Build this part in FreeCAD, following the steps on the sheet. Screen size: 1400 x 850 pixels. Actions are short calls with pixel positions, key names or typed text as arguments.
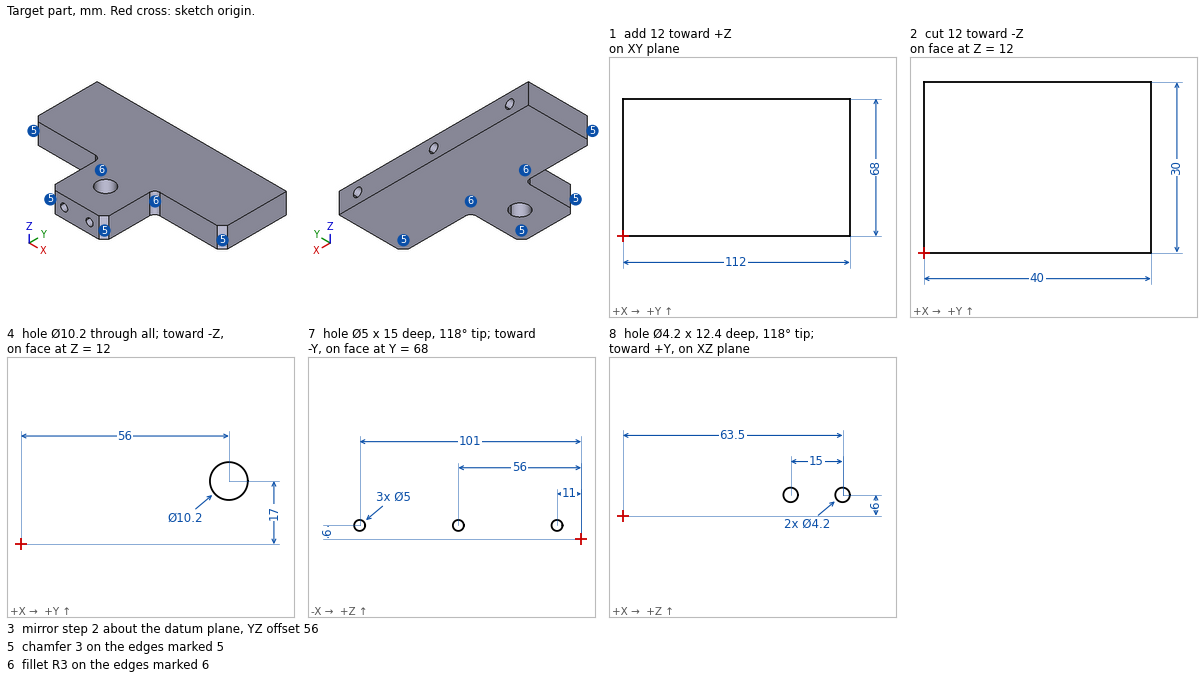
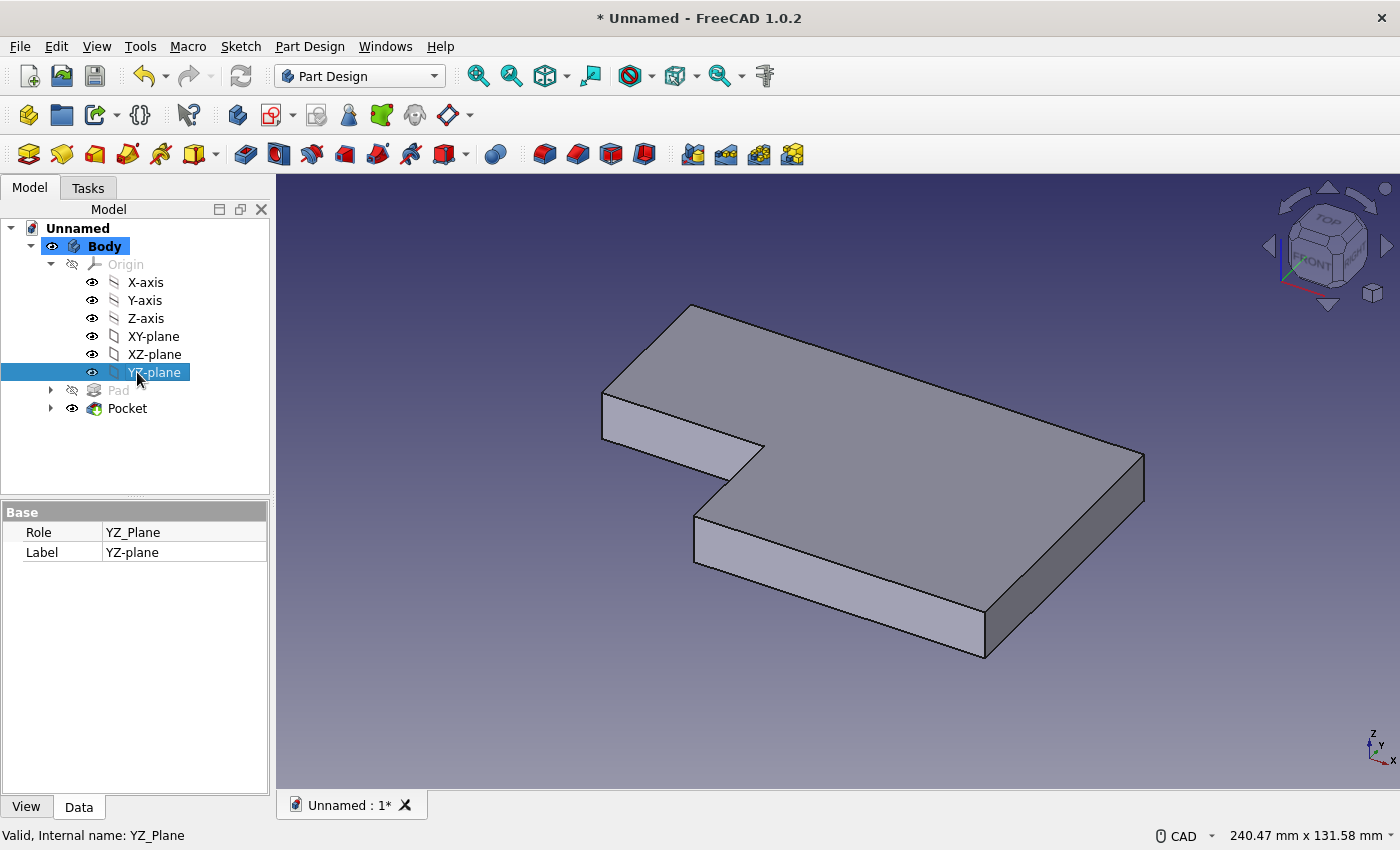
click(448, 116)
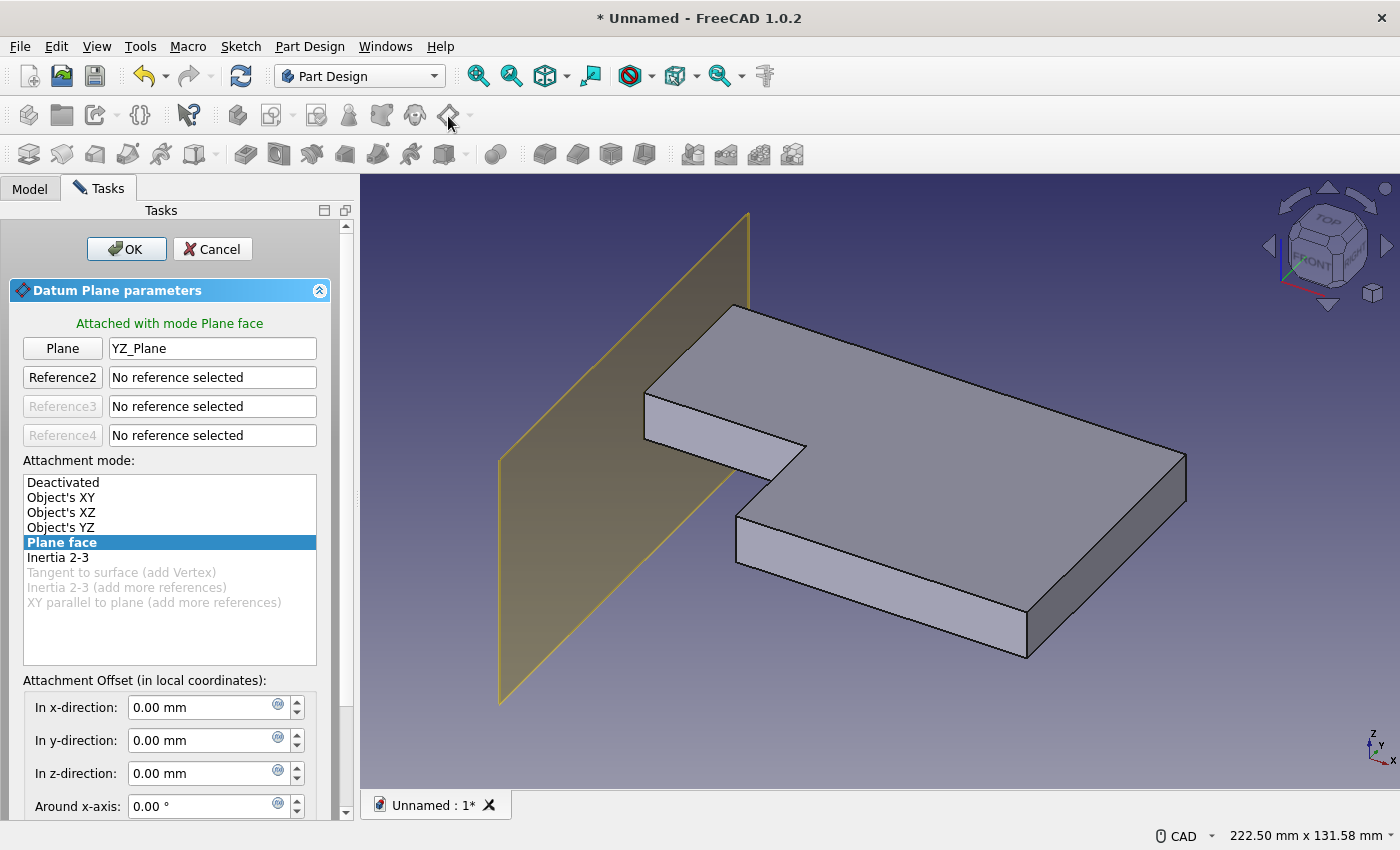
triple_click(210, 774)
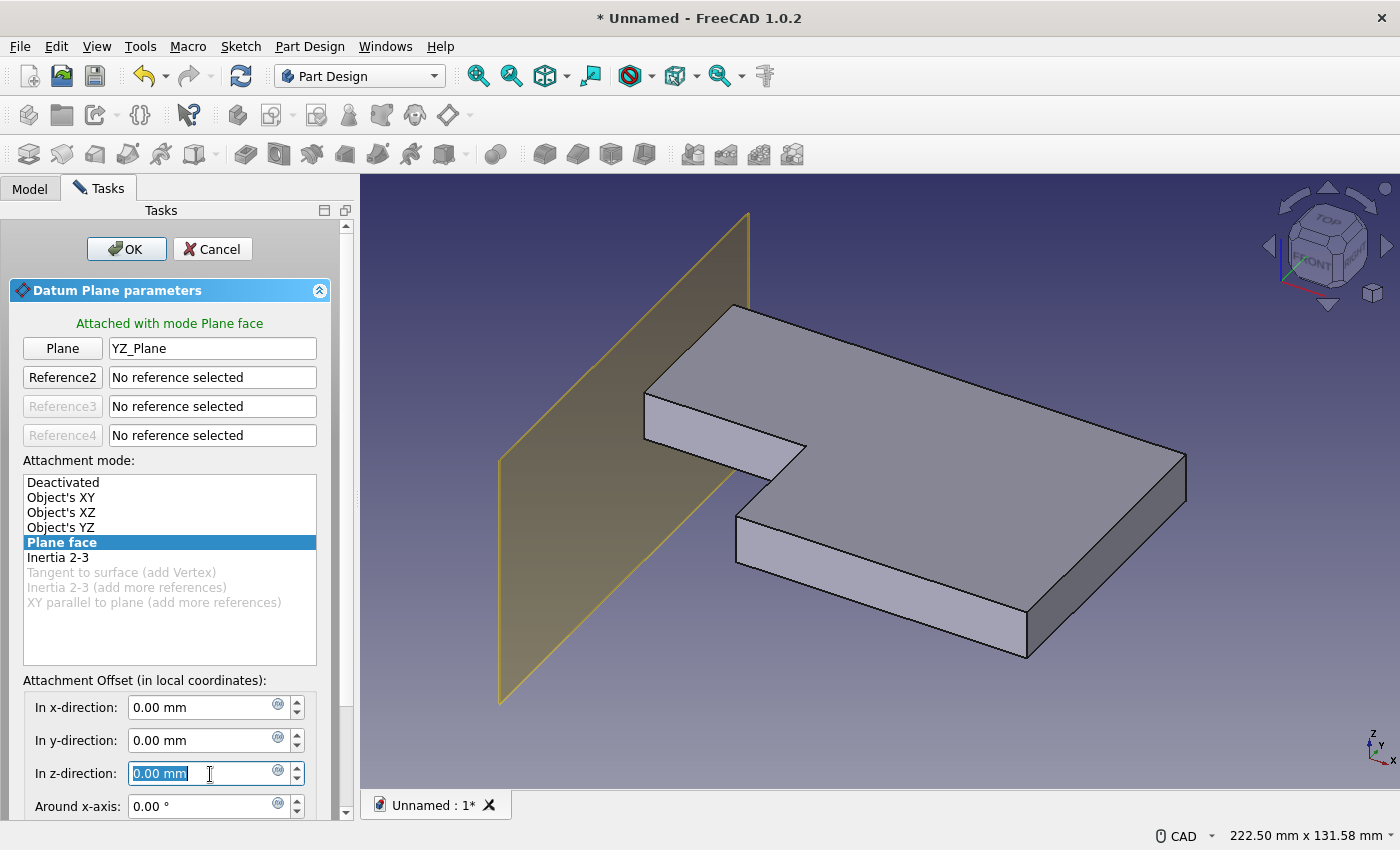
text(56)
key(Tab)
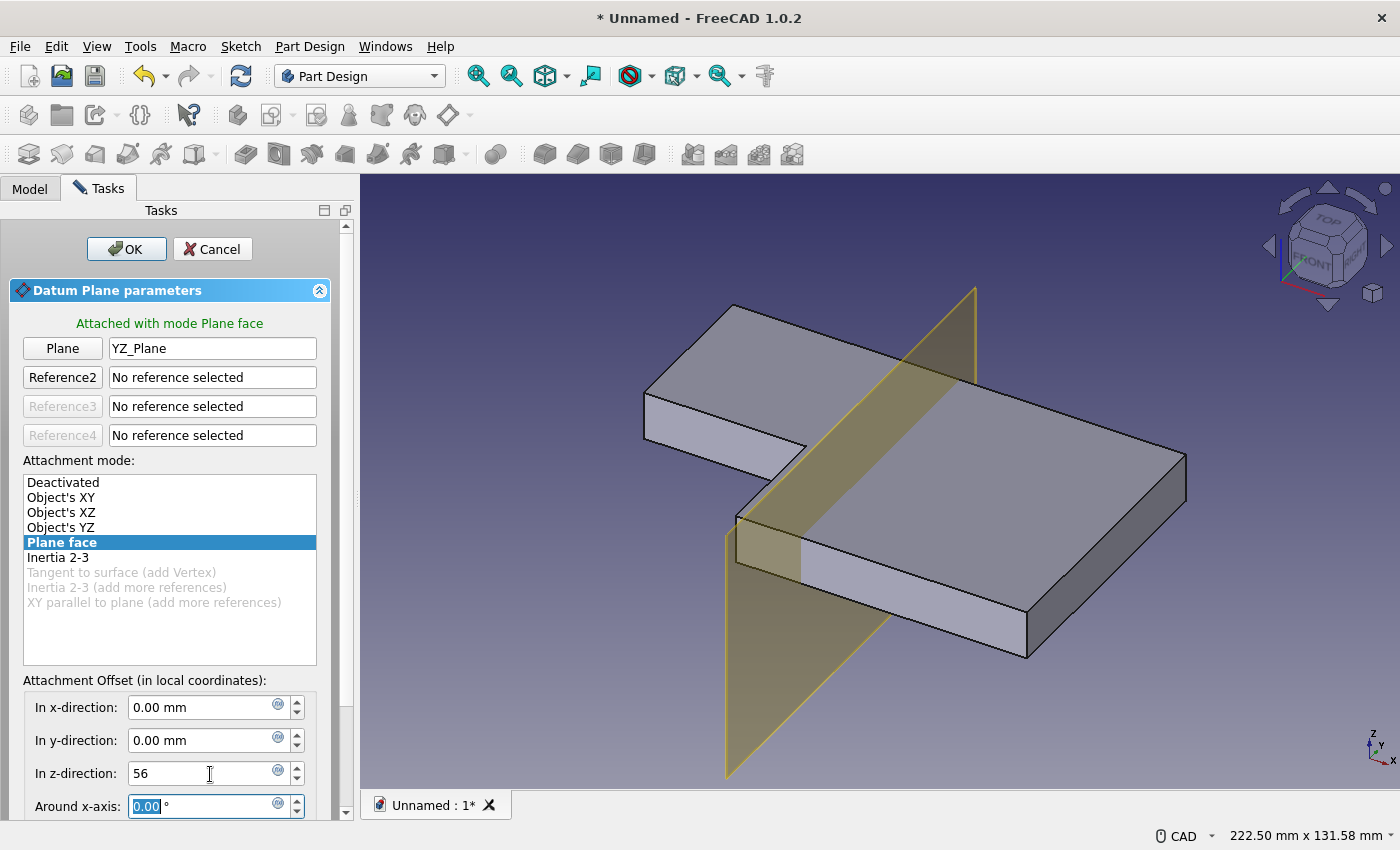
click(127, 249)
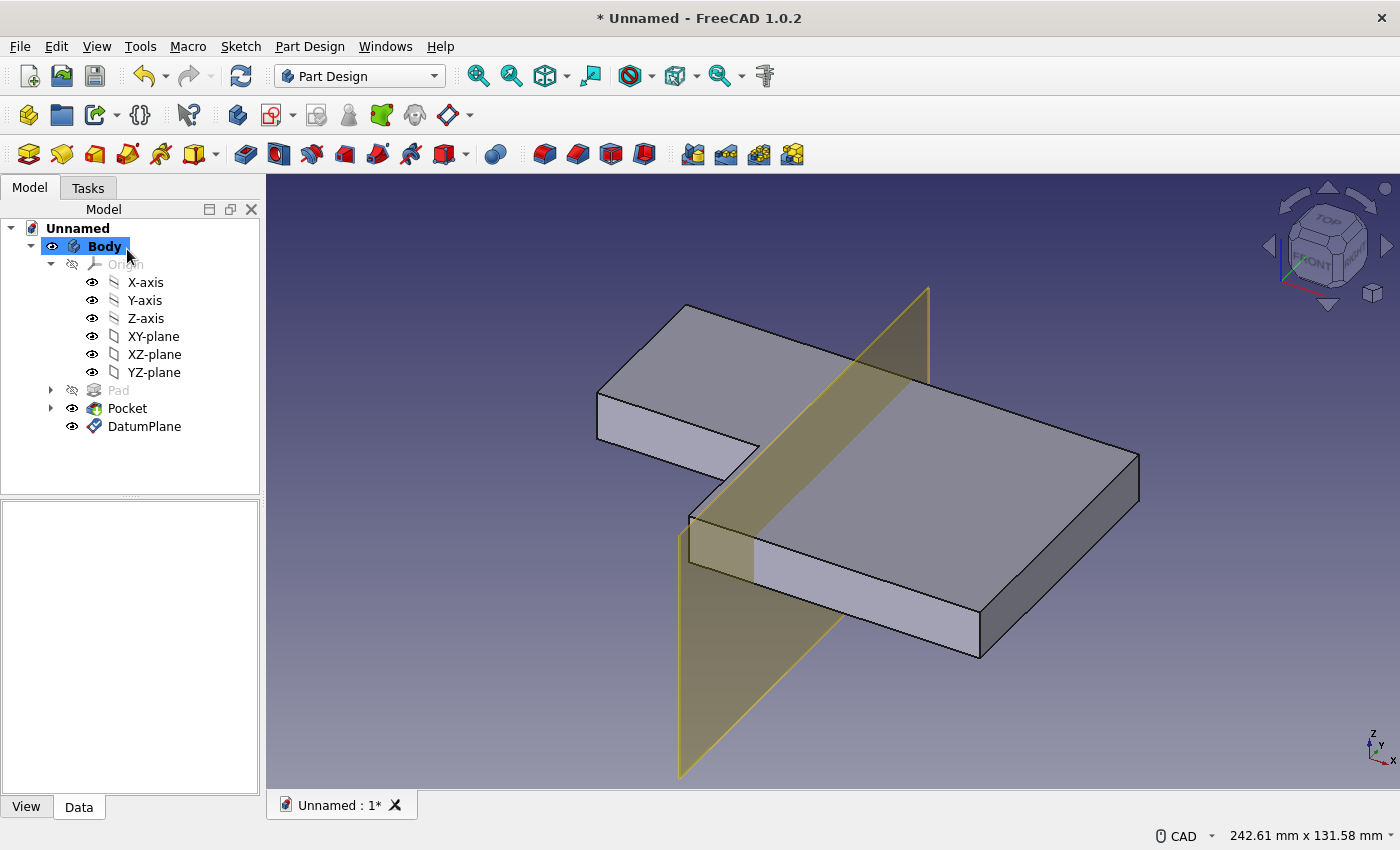
click(117, 408)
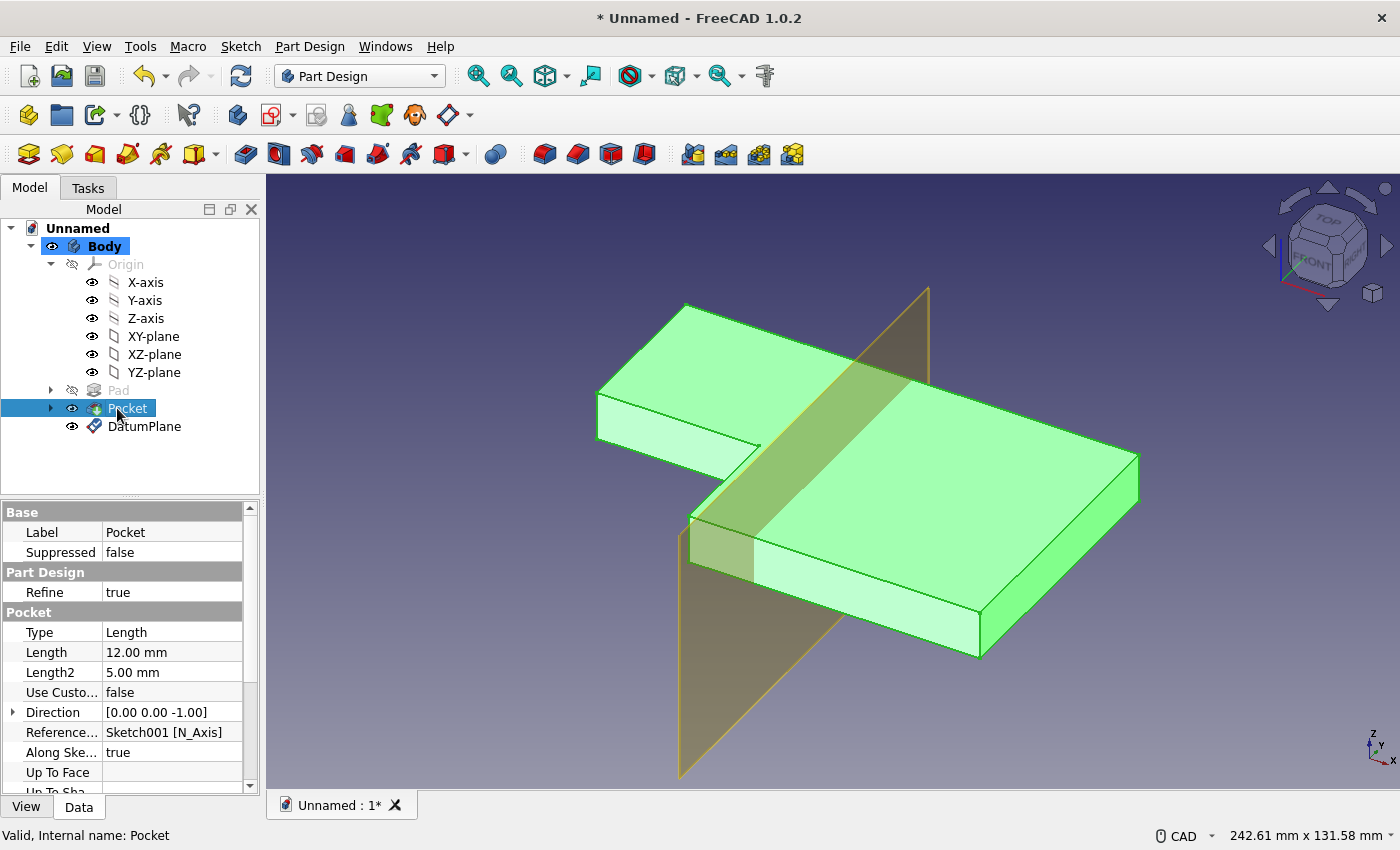
click(693, 154)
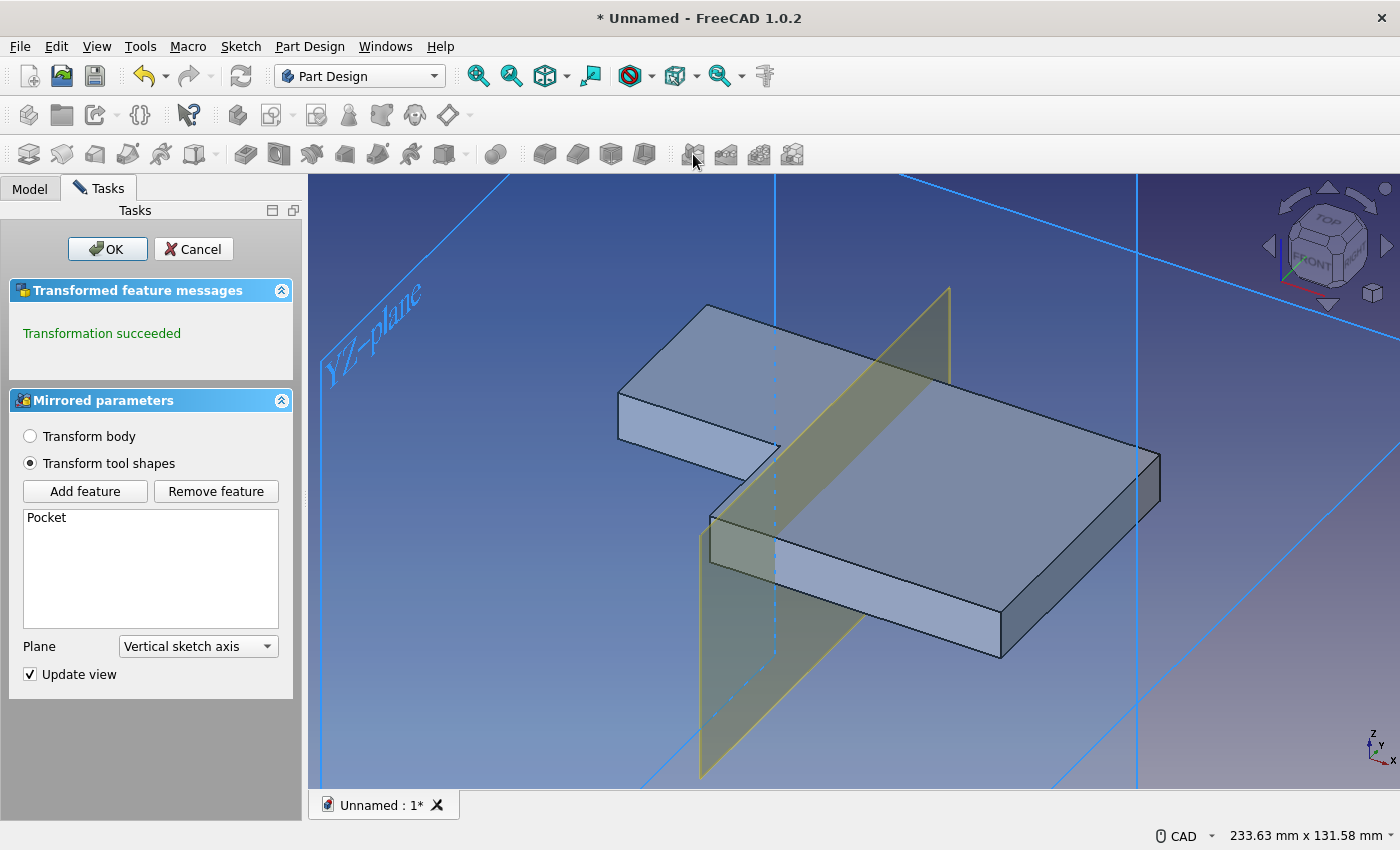
click(199, 646)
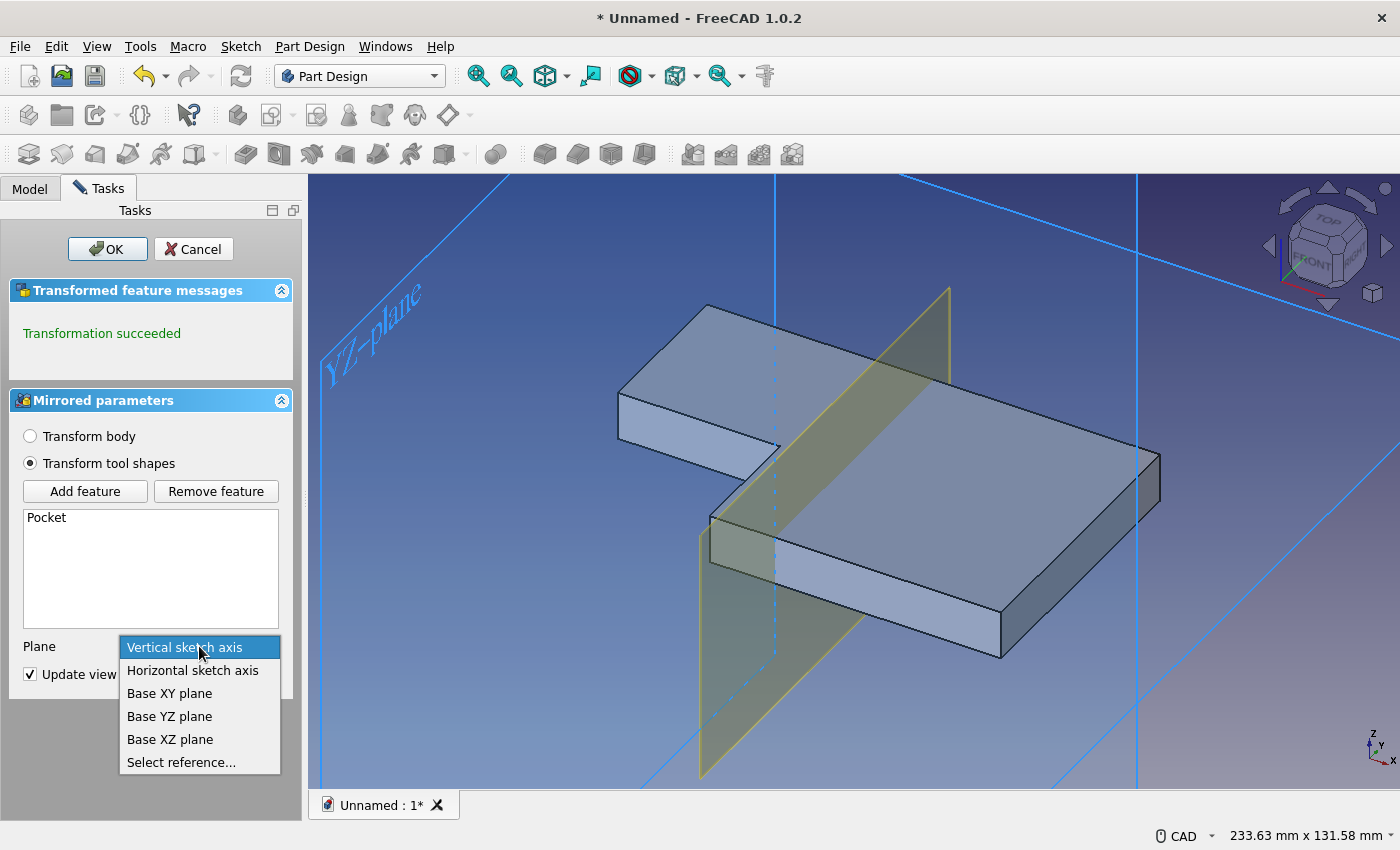
click(198, 762)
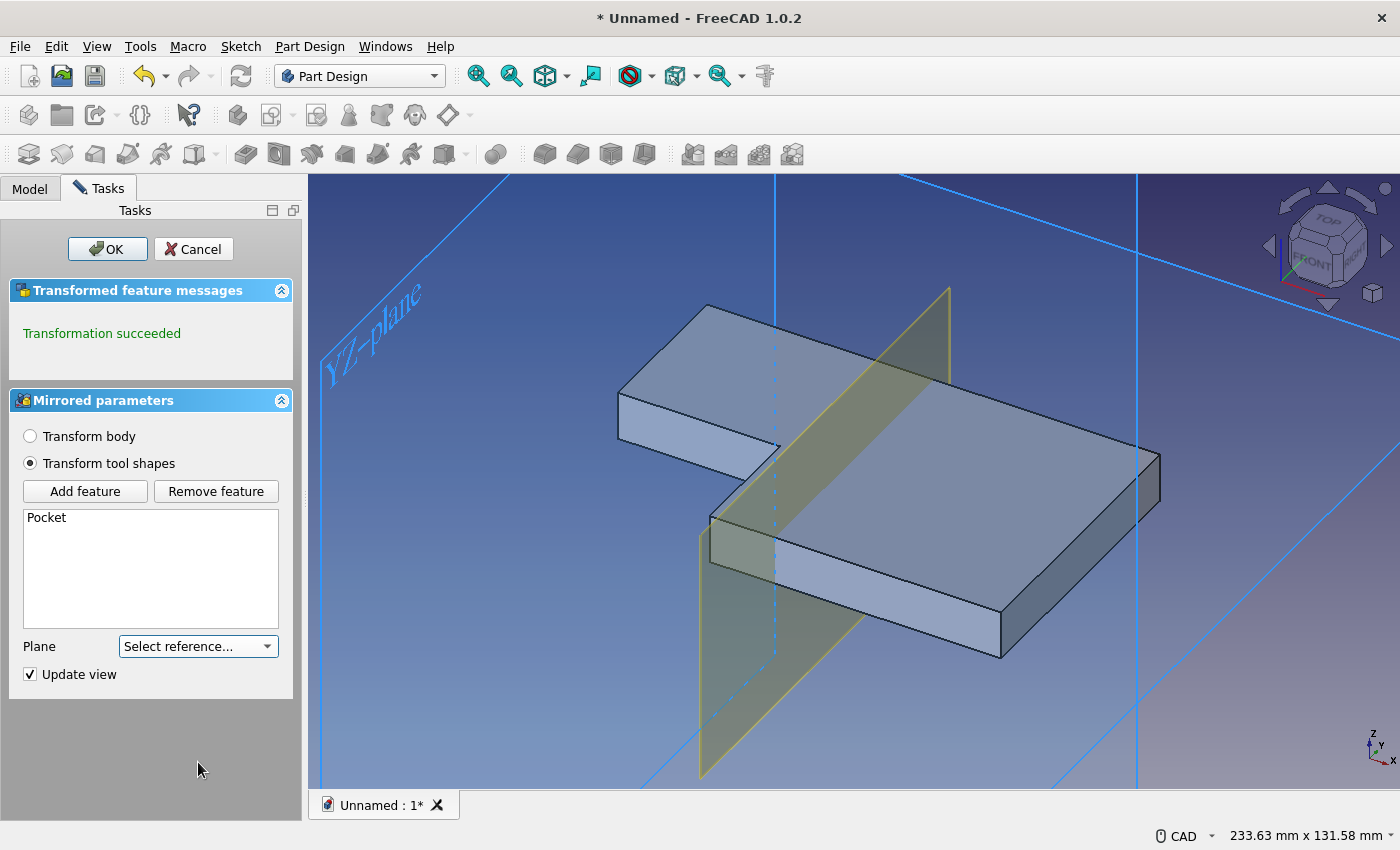
click(30, 188)